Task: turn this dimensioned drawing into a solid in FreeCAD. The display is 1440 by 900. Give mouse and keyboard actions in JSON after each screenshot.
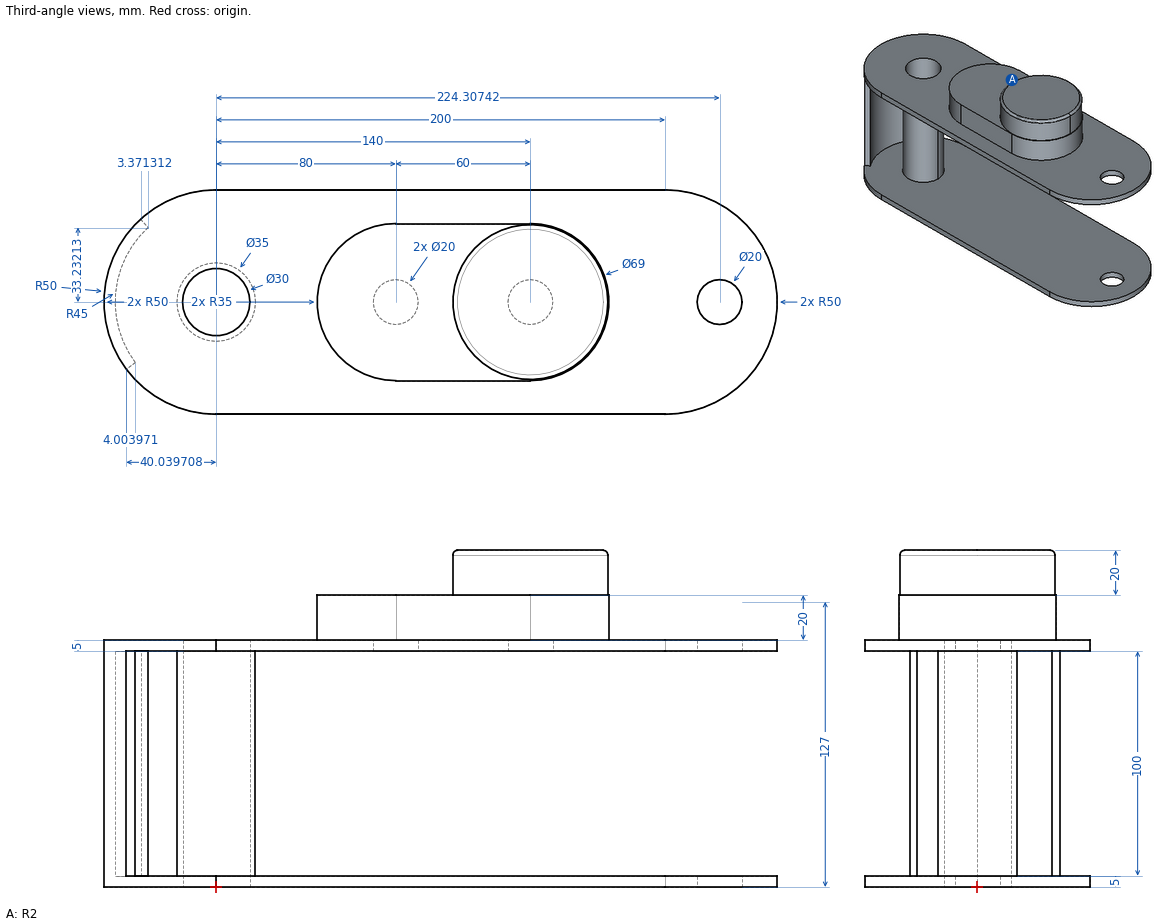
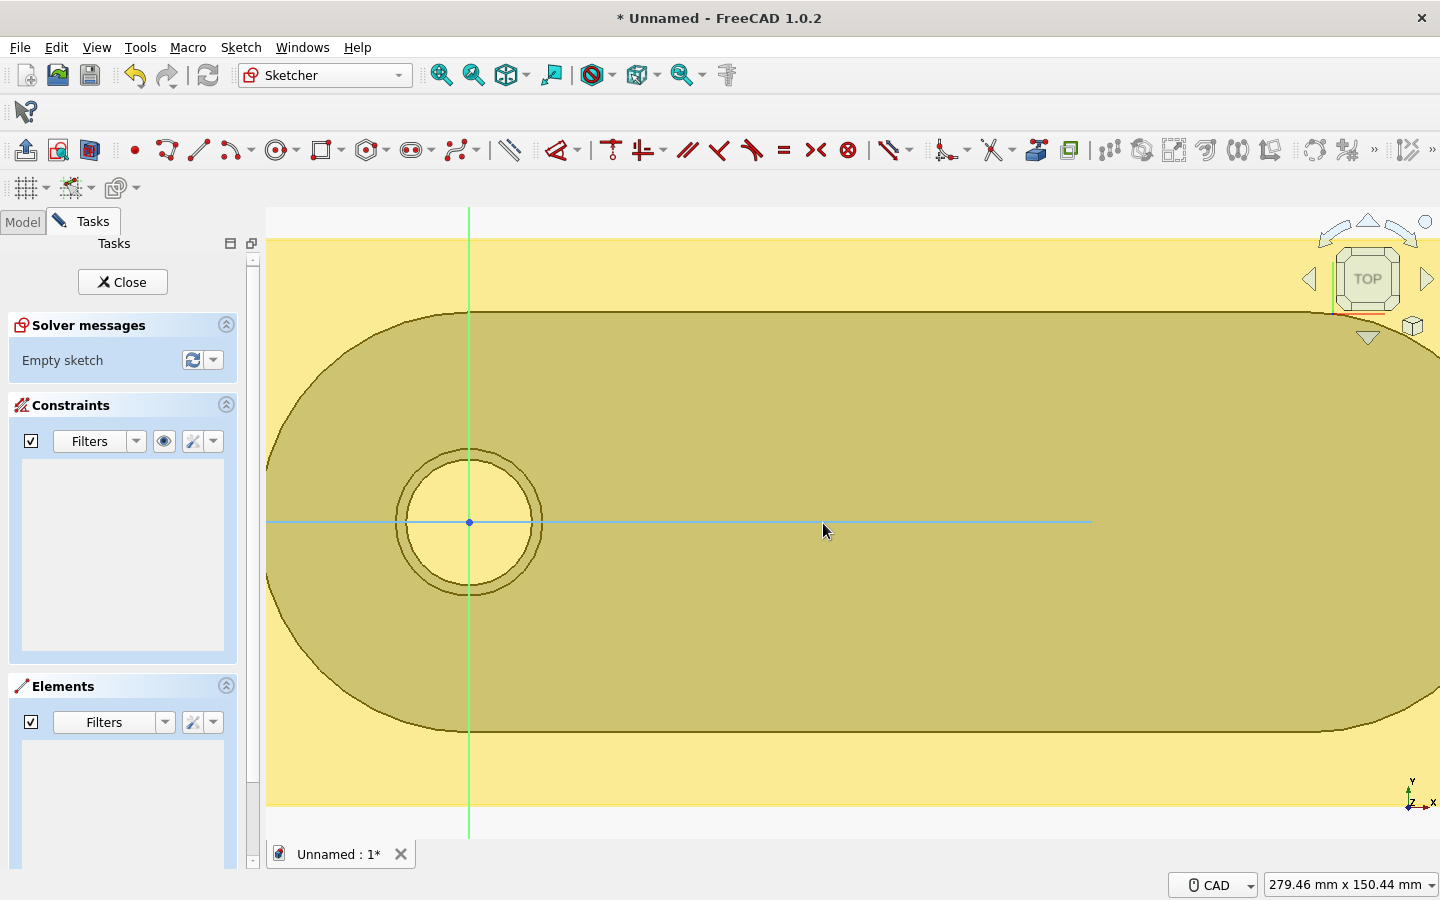
{"action": "left_click", "coordinate": [276, 150]}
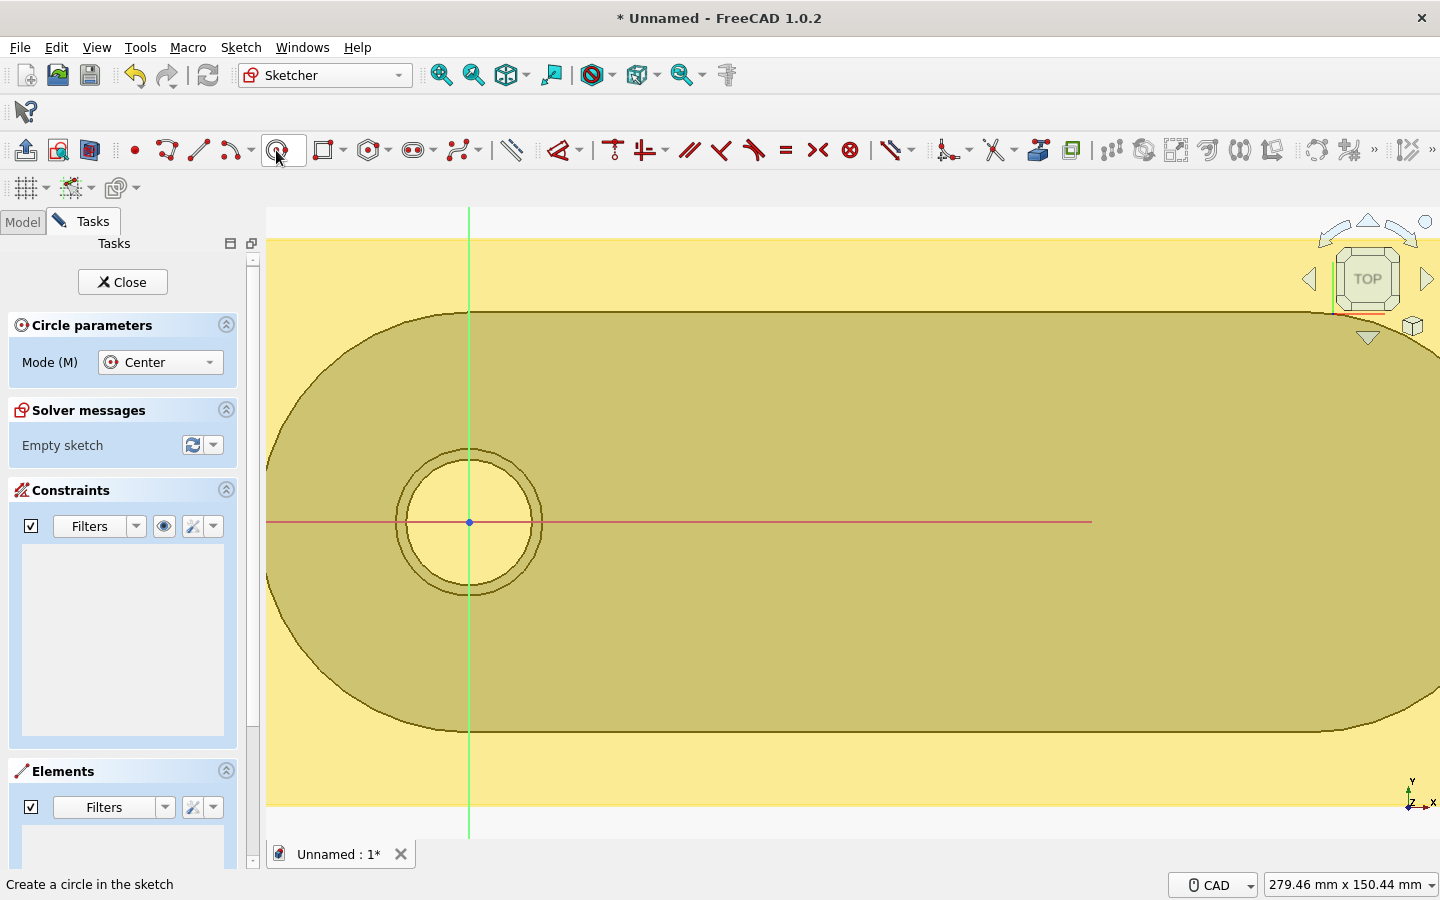
{"action": "left_click", "coordinate": [805, 522]}
{"action": "left_click", "coordinate": [835, 493]}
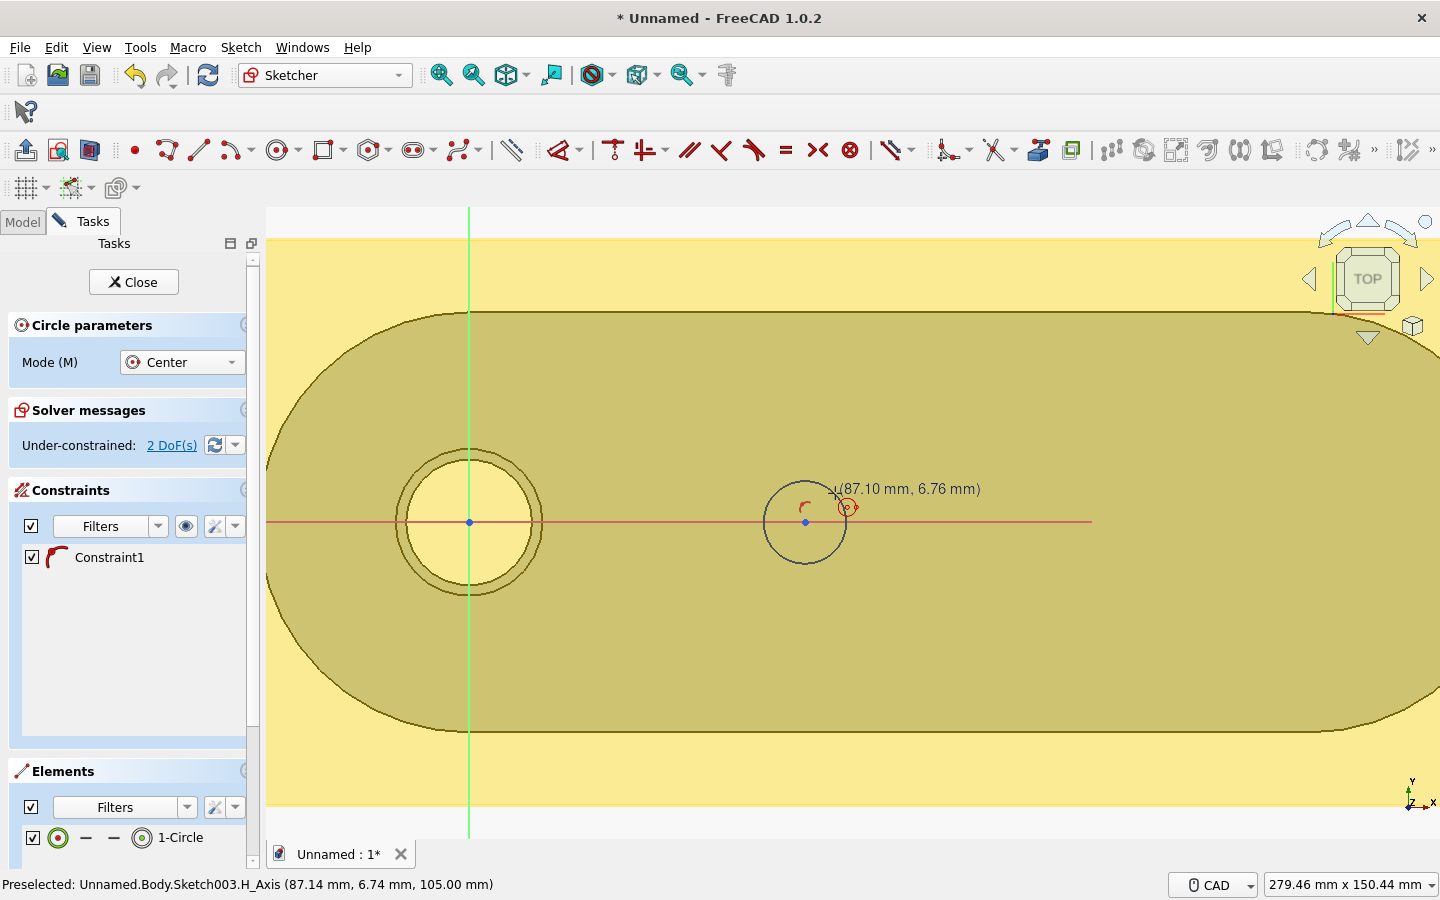
{"action": "left_click", "coordinate": [1057, 522]}
{"action": "left_click", "coordinate": [1087, 493]}
{"action": "key", "text": "Escape"}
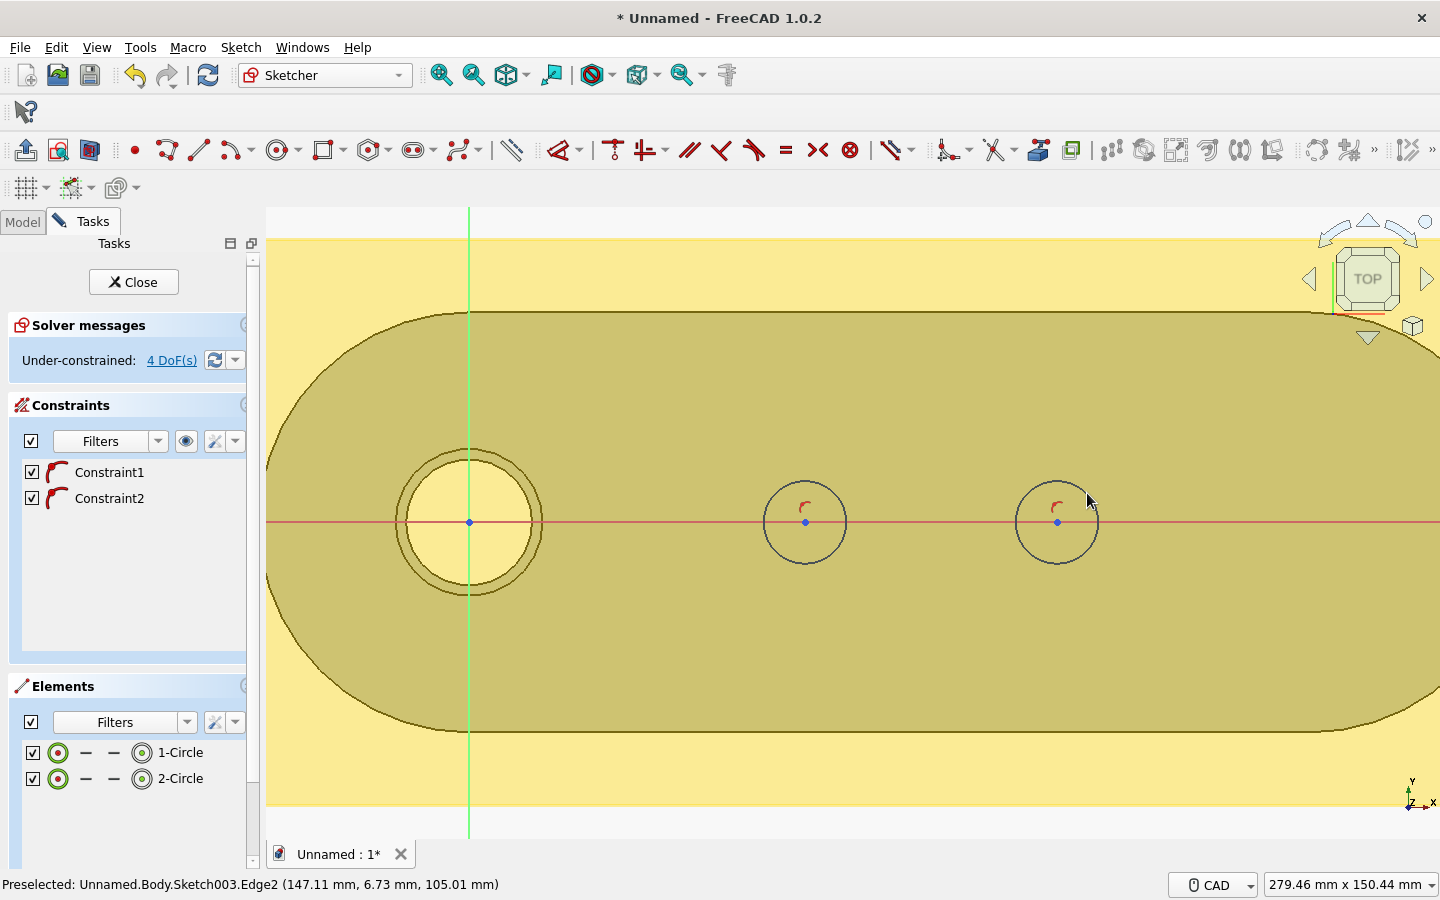
{"action": "left_click", "coordinate": [834, 493]}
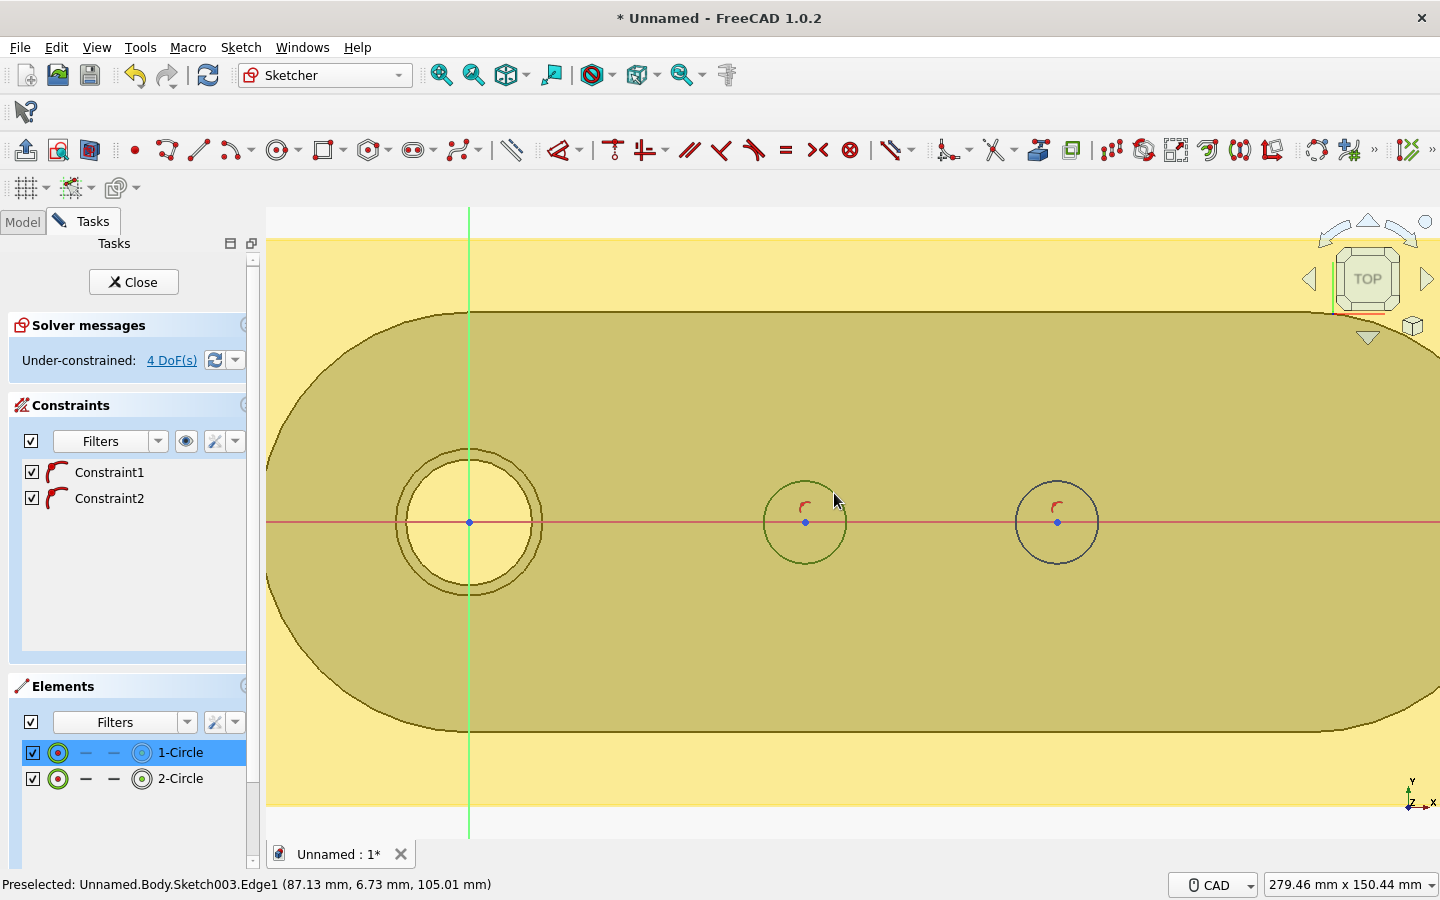
{"action": "left_click", "coordinate": [1086, 493]}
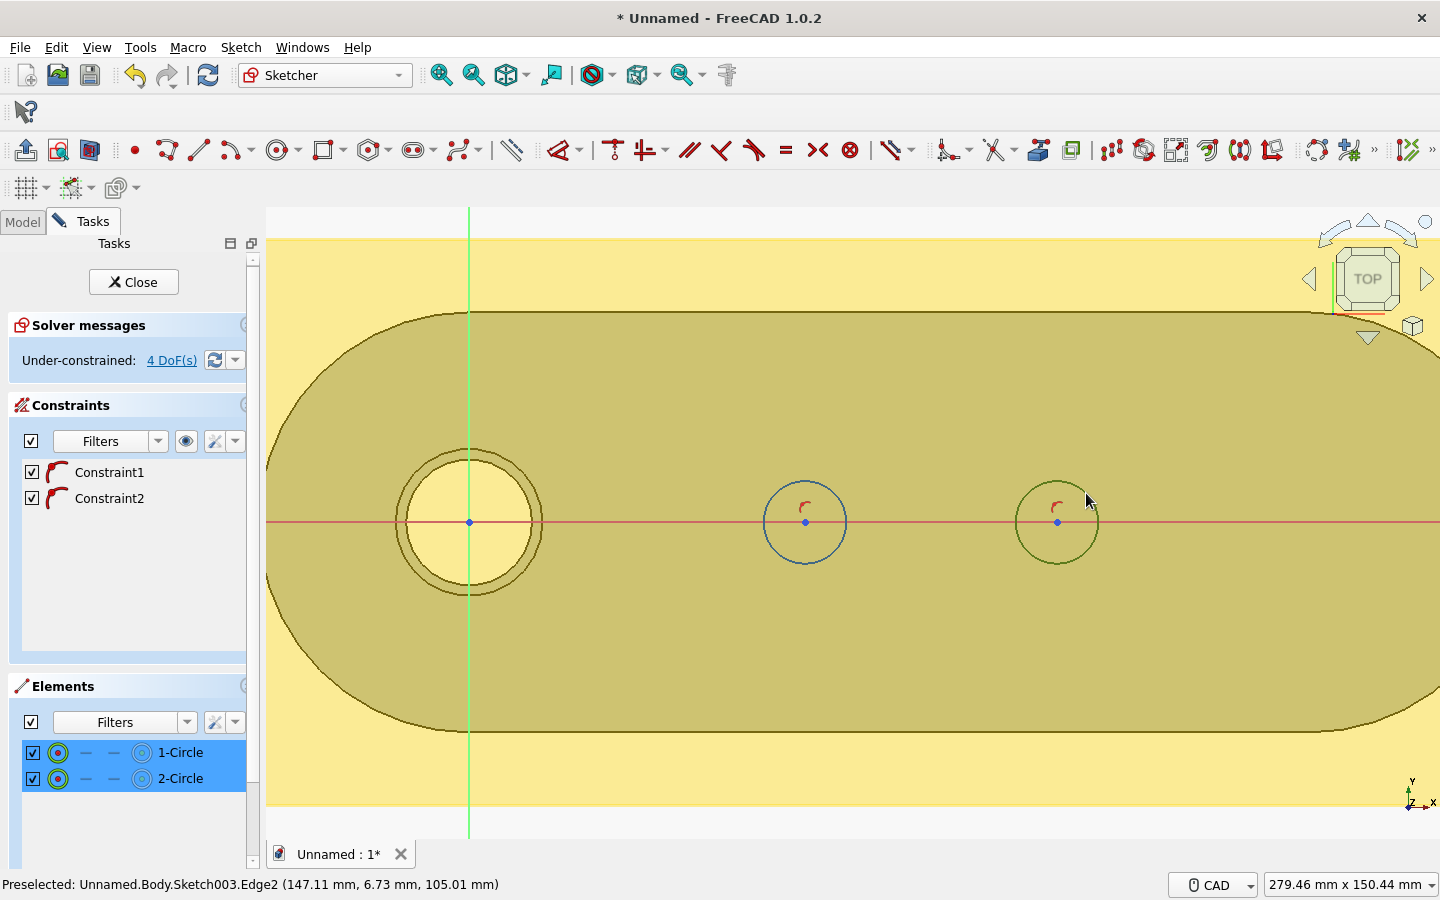
{"action": "left_click", "coordinate": [786, 150]}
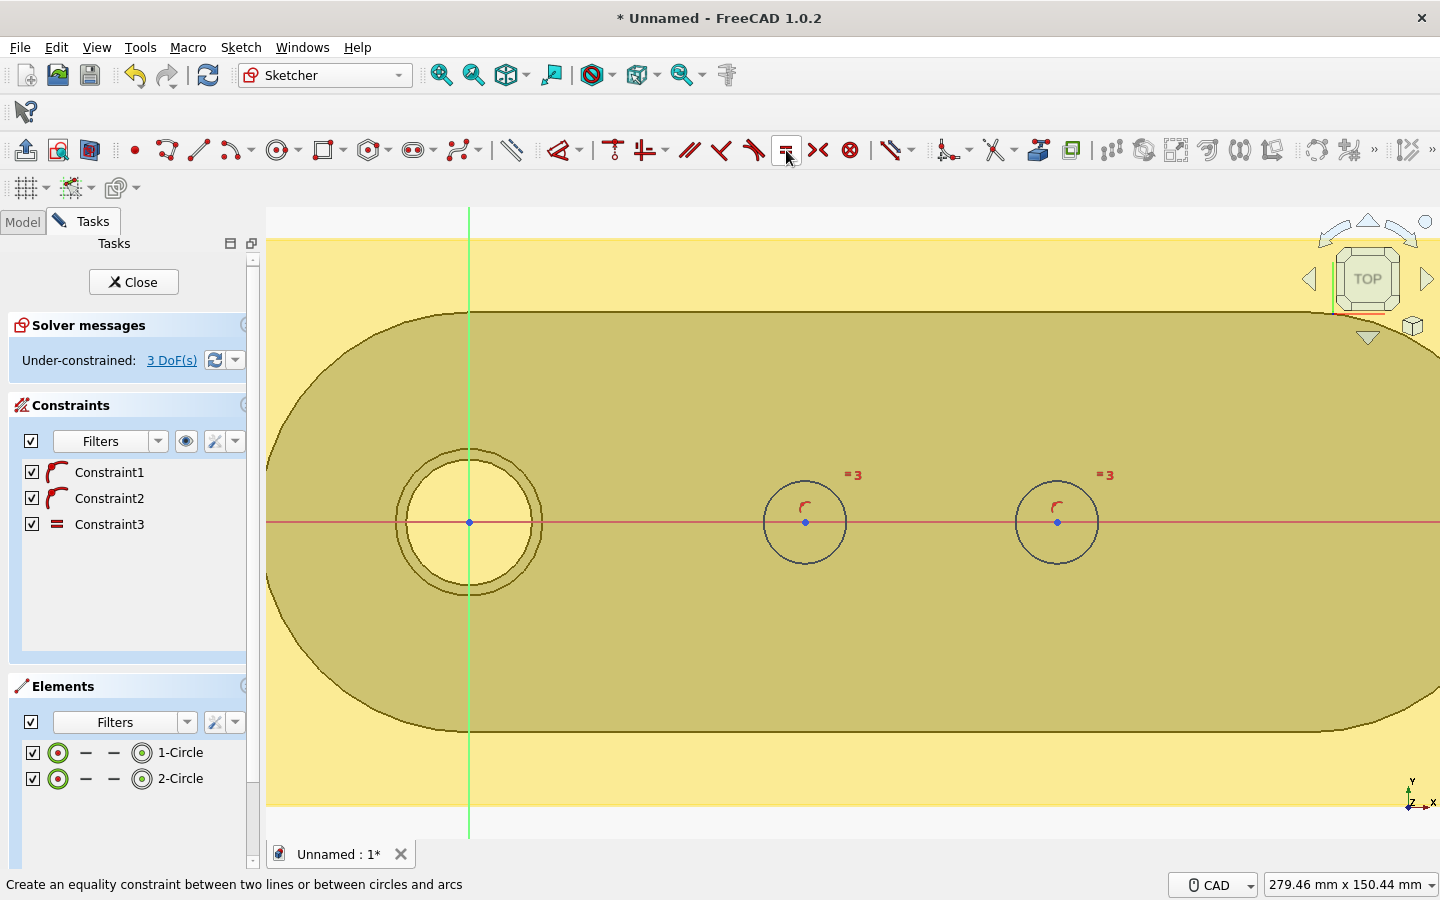
{"action": "left_click", "coordinate": [558, 150]}